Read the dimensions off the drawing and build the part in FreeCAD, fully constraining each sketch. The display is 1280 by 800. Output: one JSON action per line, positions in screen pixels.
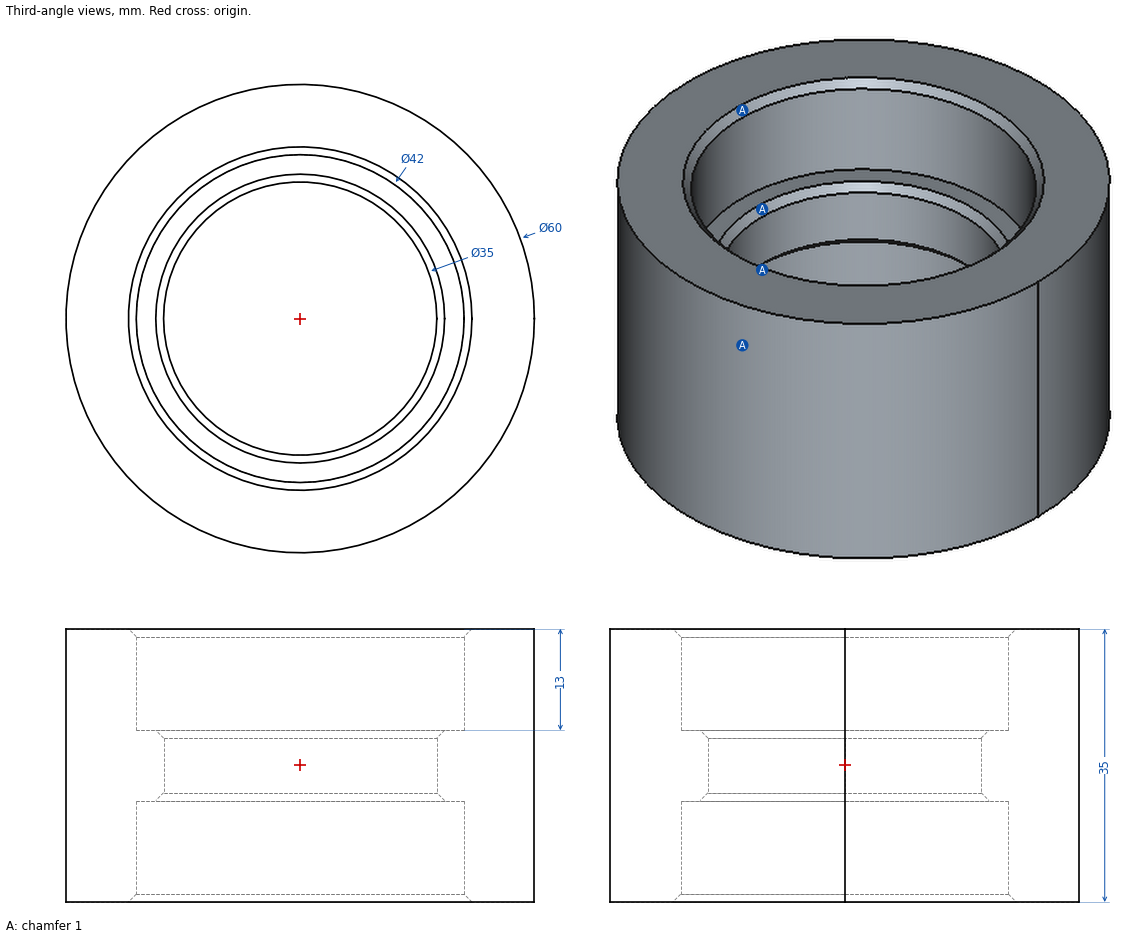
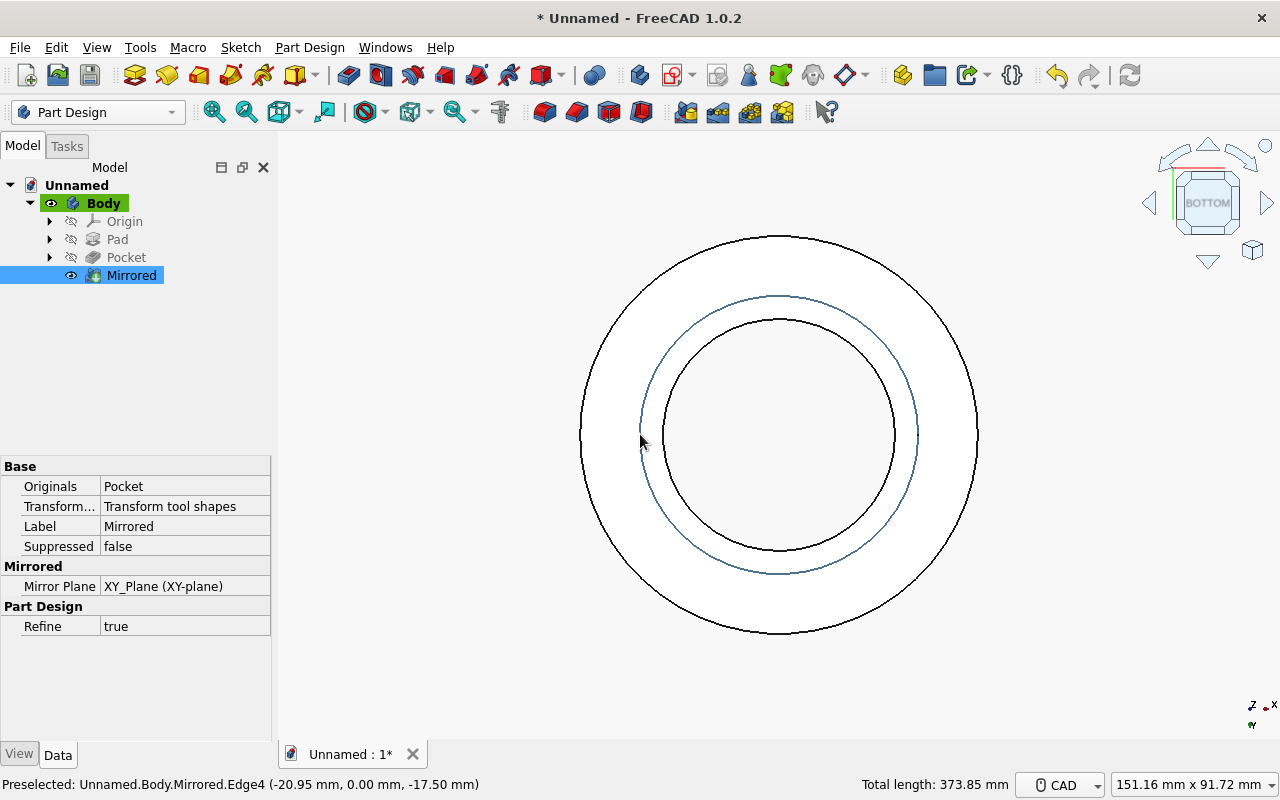
{"action": "left_click", "coordinate": [663, 434], "text": "ctrl"}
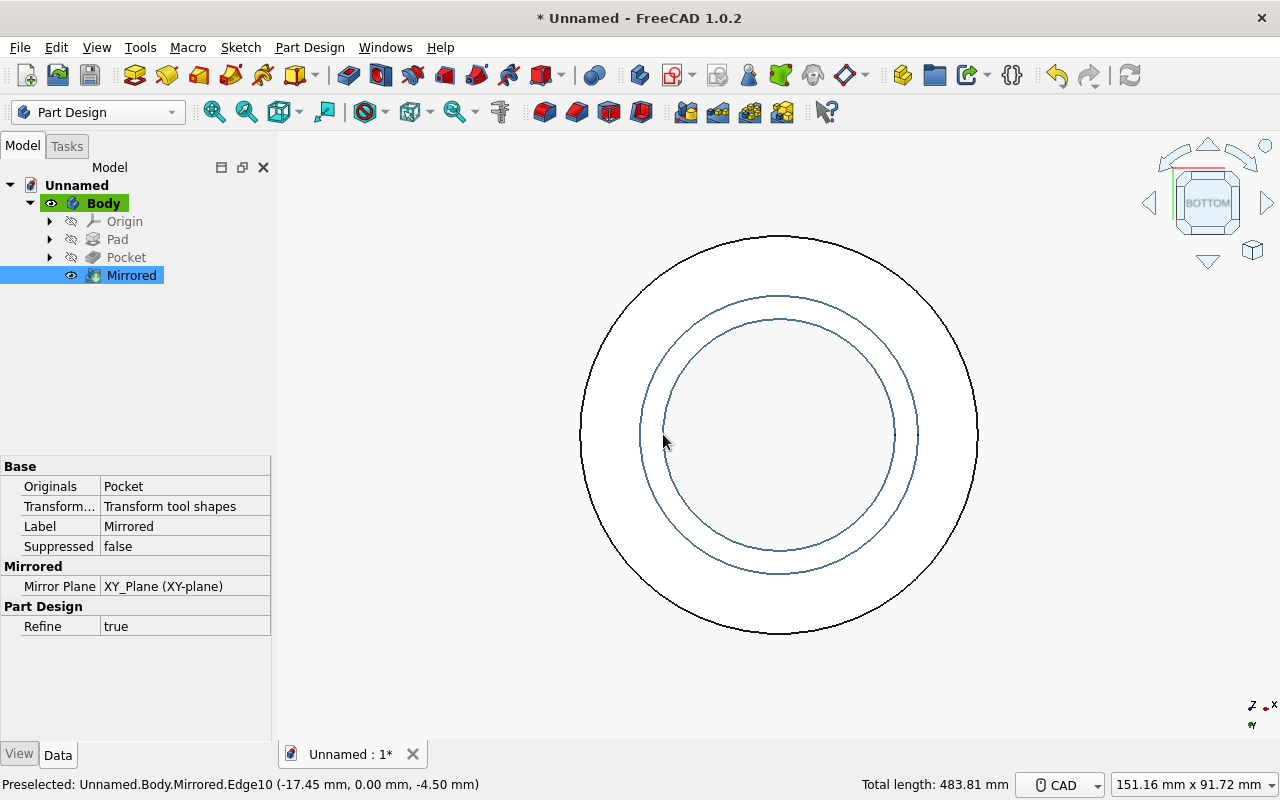
{"action": "left_click", "coordinate": [578, 112]}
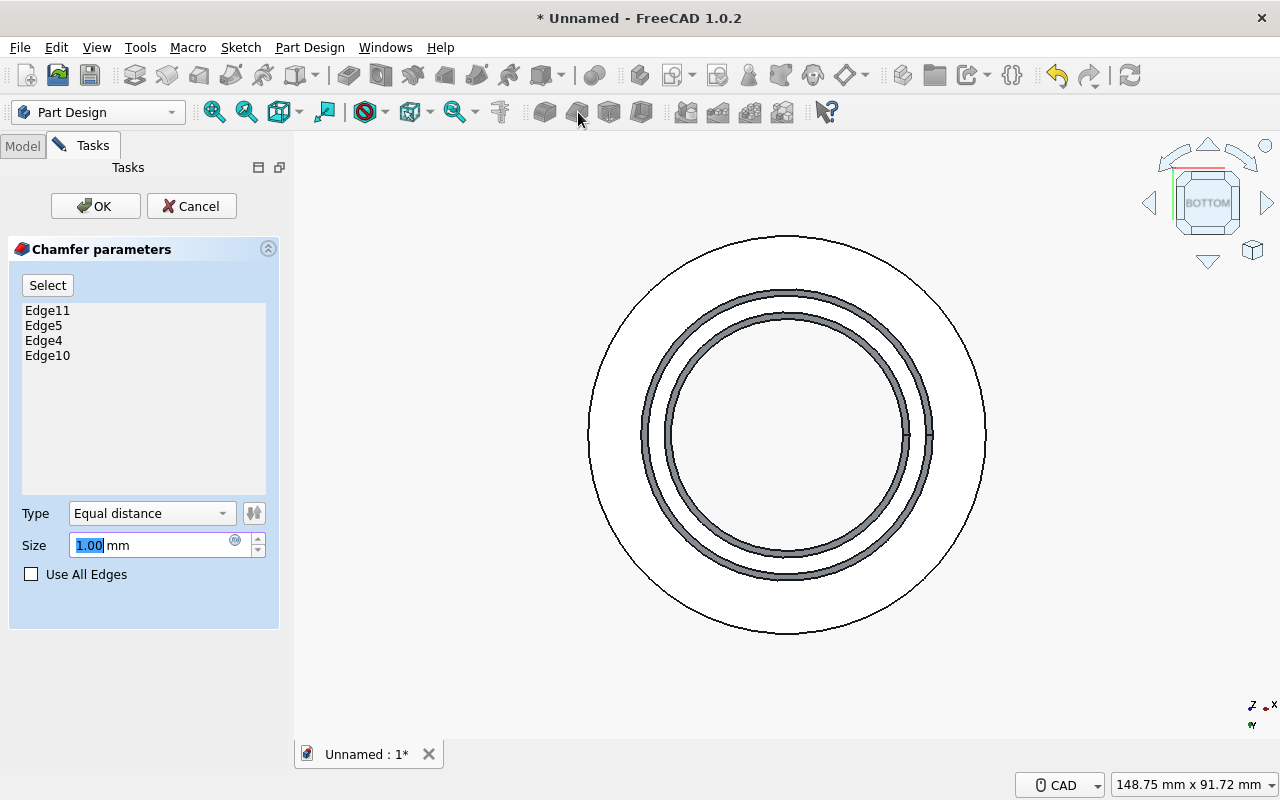
{"action": "type", "text": "1"}
{"action": "key", "text": "Tab"}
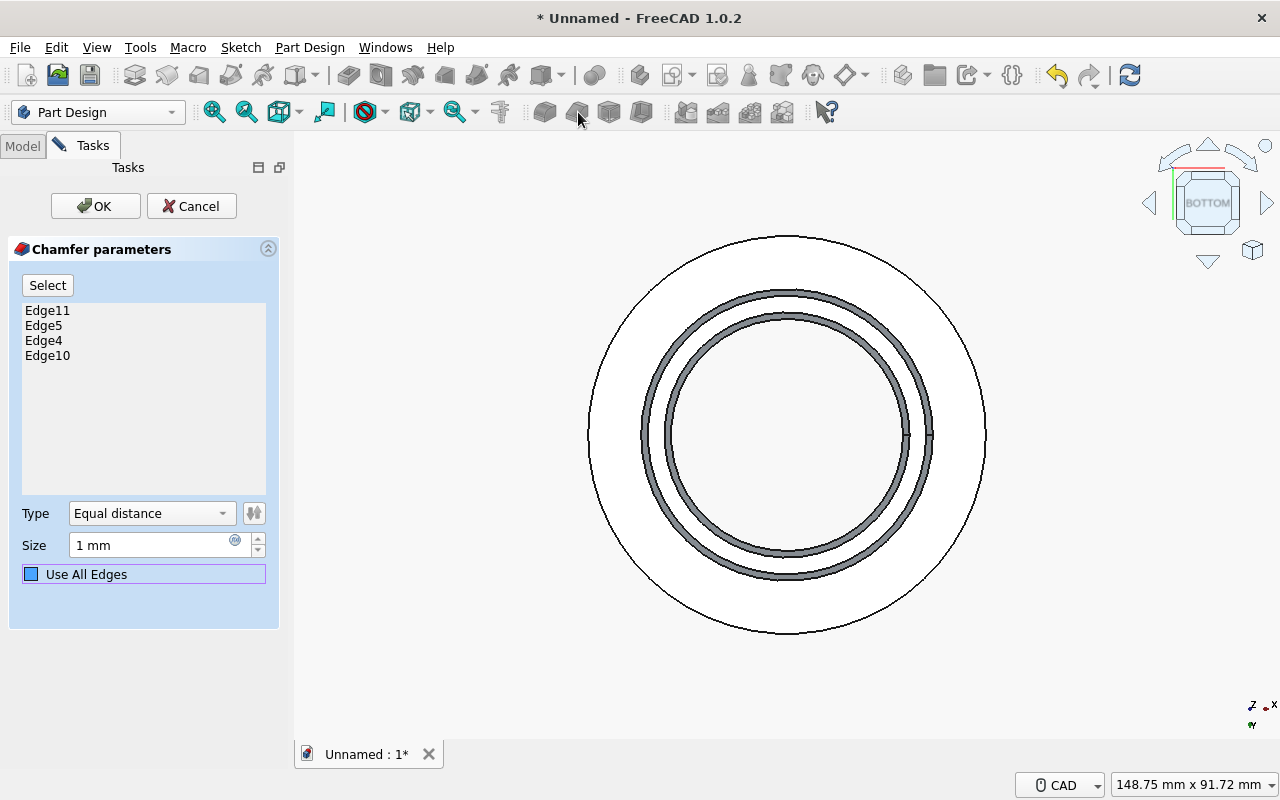
{"action": "left_click", "coordinate": [96, 206]}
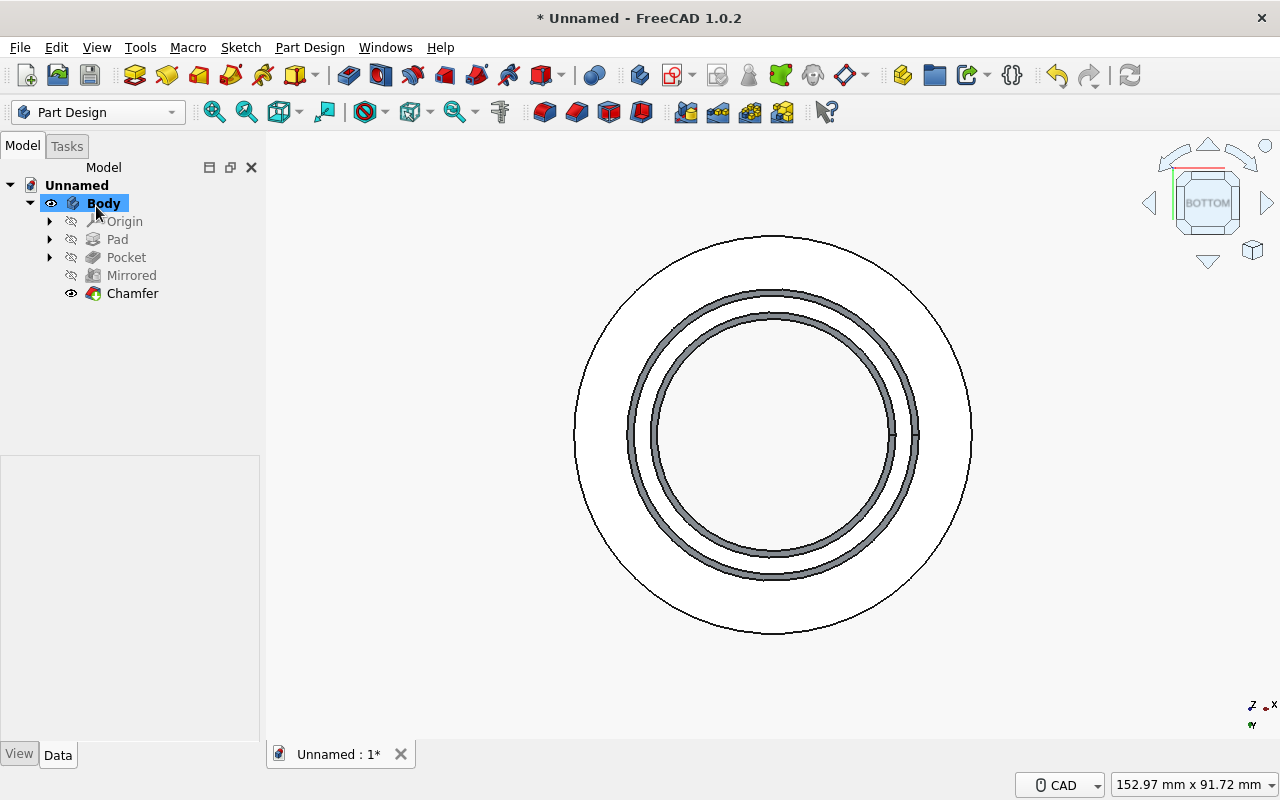
{"action": "key", "text": "0"}